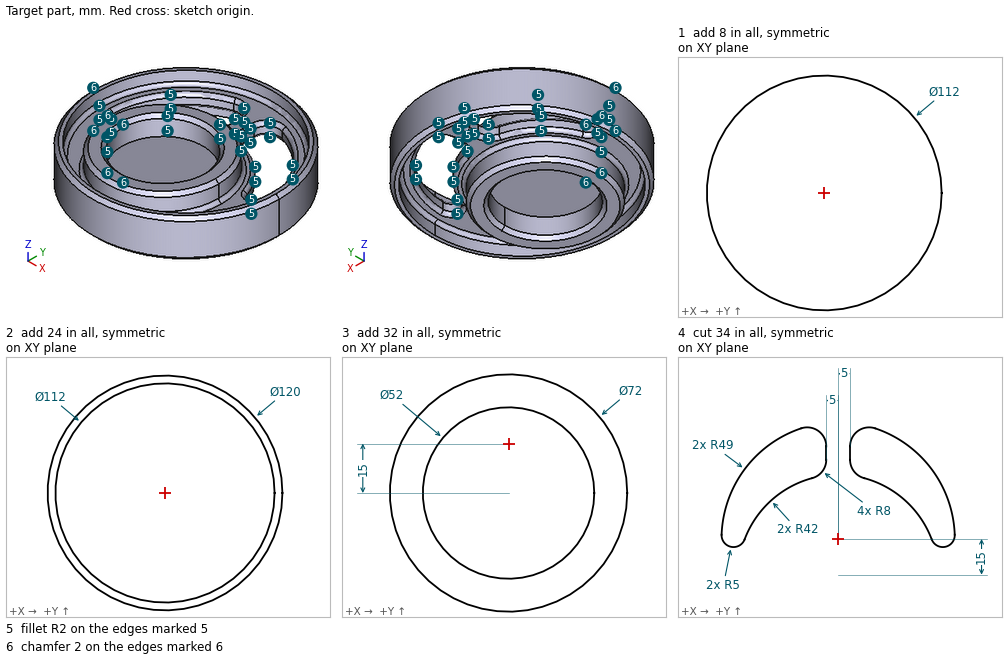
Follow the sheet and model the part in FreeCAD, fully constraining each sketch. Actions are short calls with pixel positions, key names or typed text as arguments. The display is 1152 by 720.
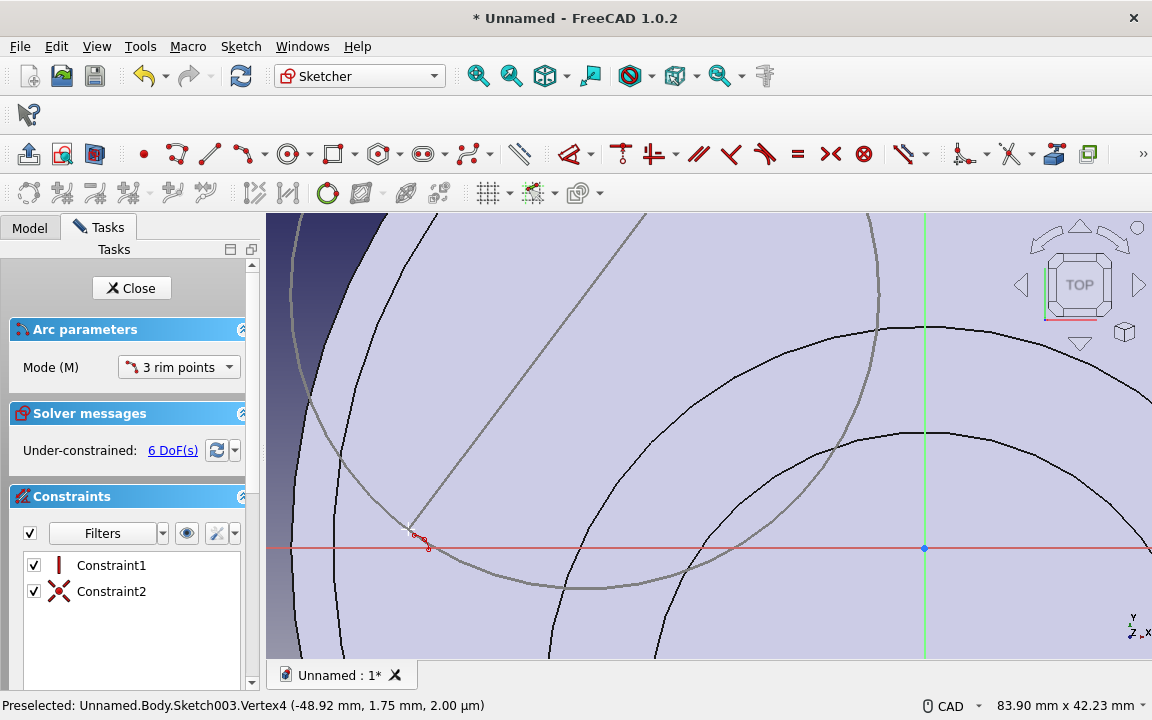
scroll(409, 530, down, 4)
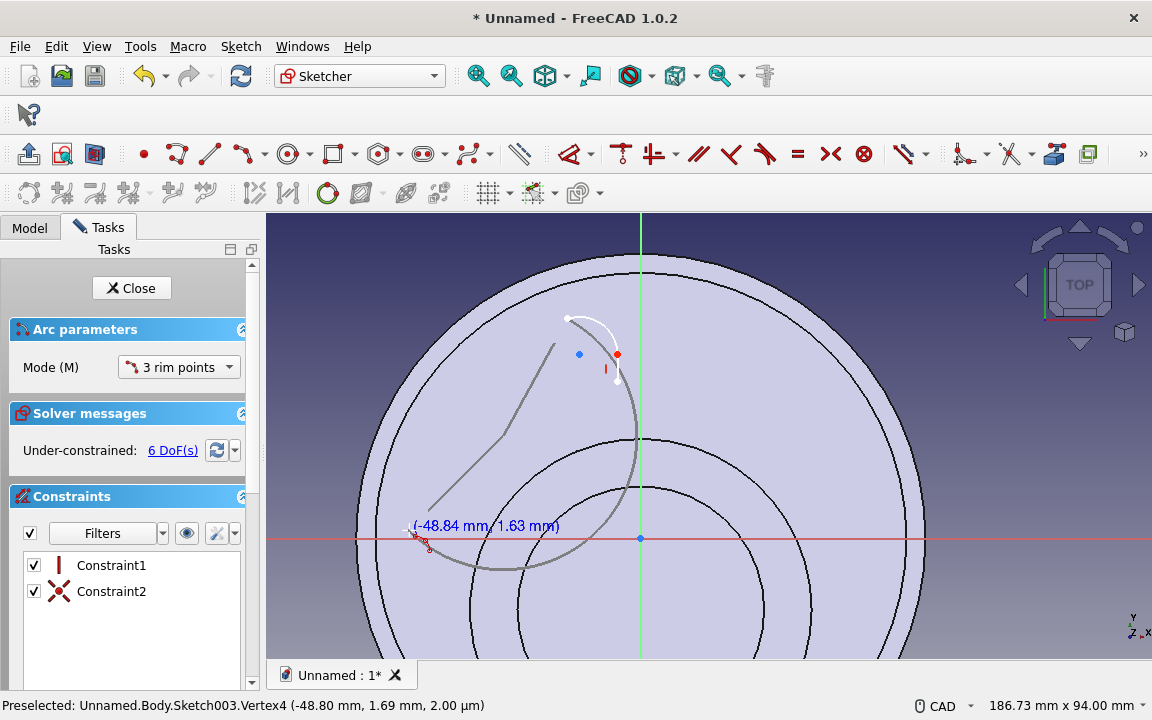
click(455, 399)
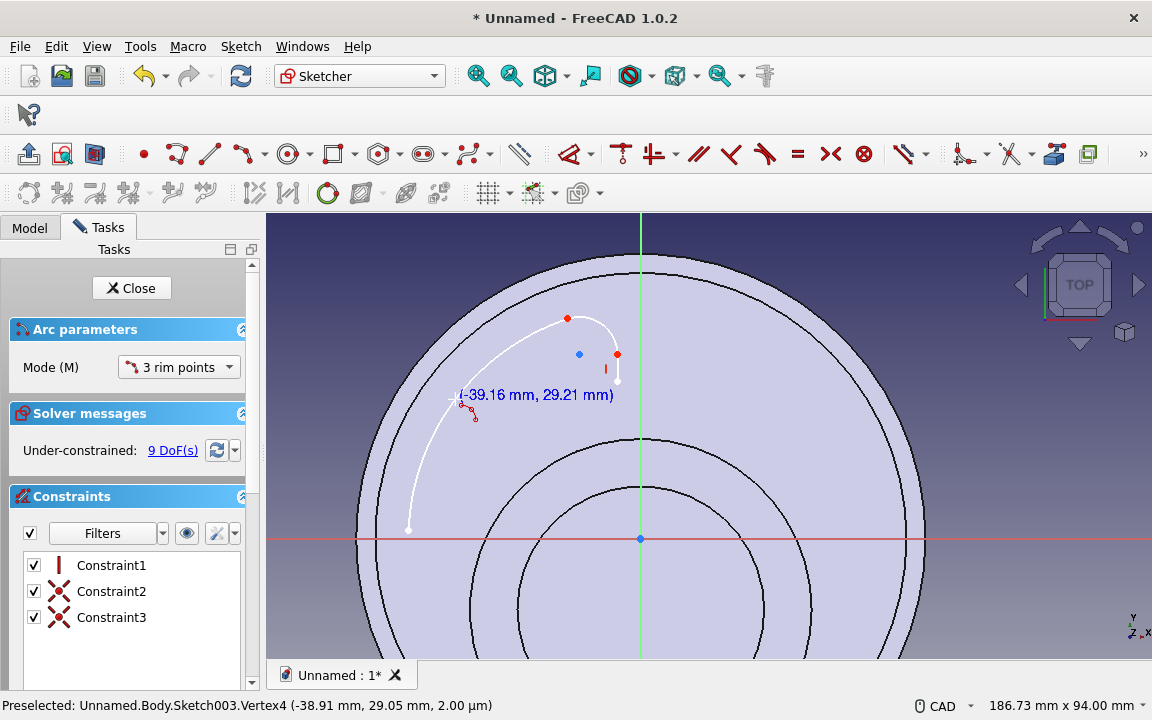
scroll(408, 530, up, 4)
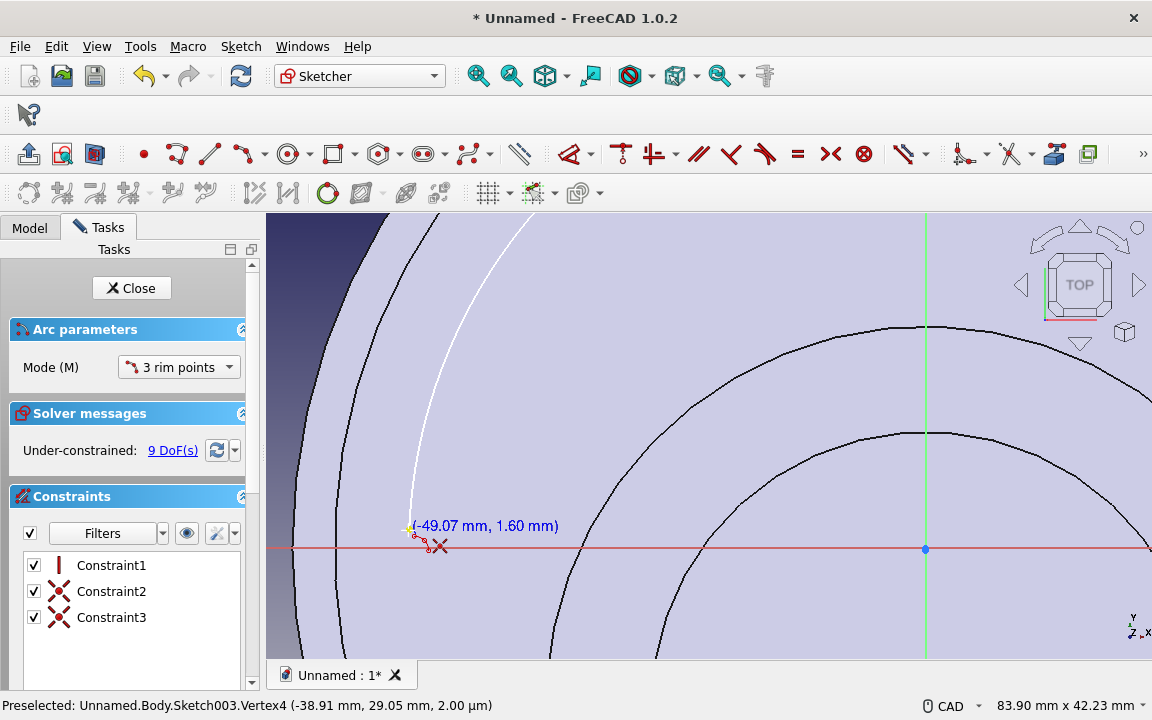
click(409, 530)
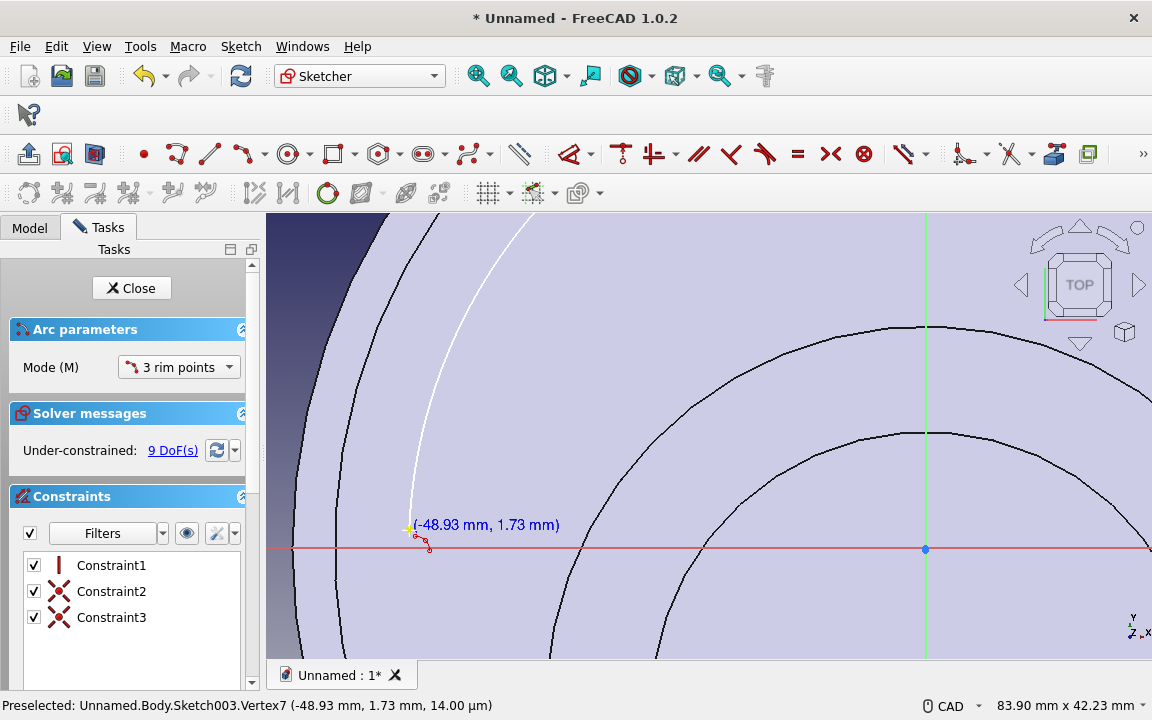
scroll(511, 550, up, 12)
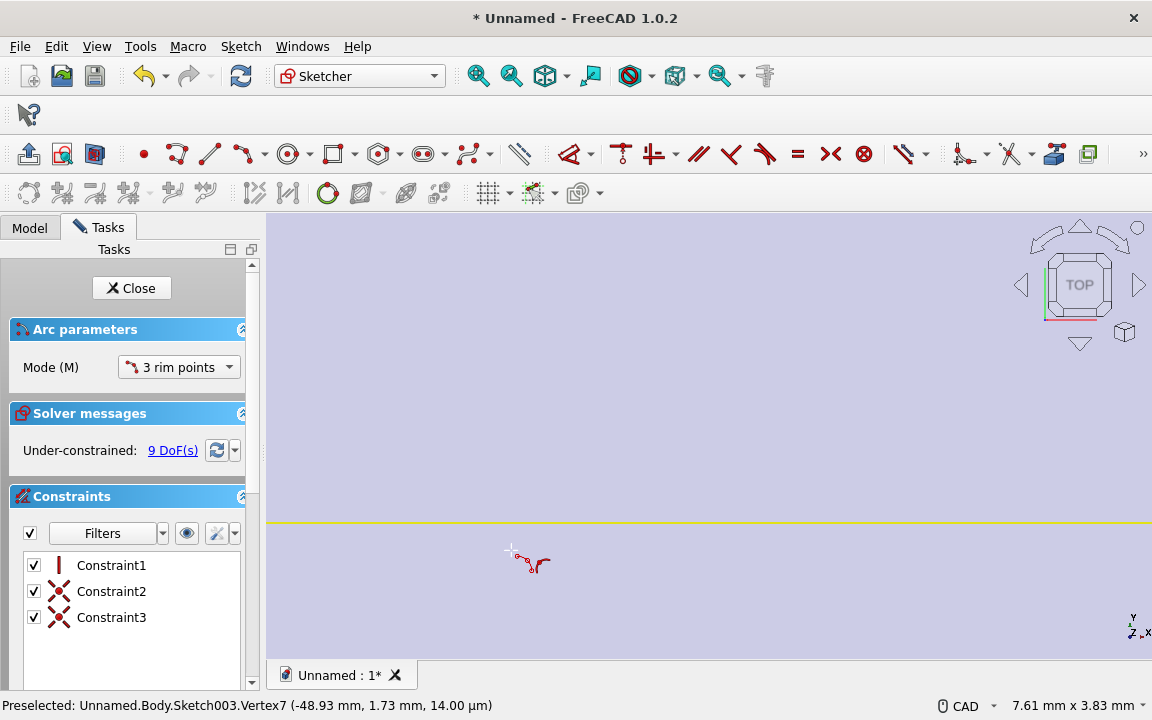
click(509, 542)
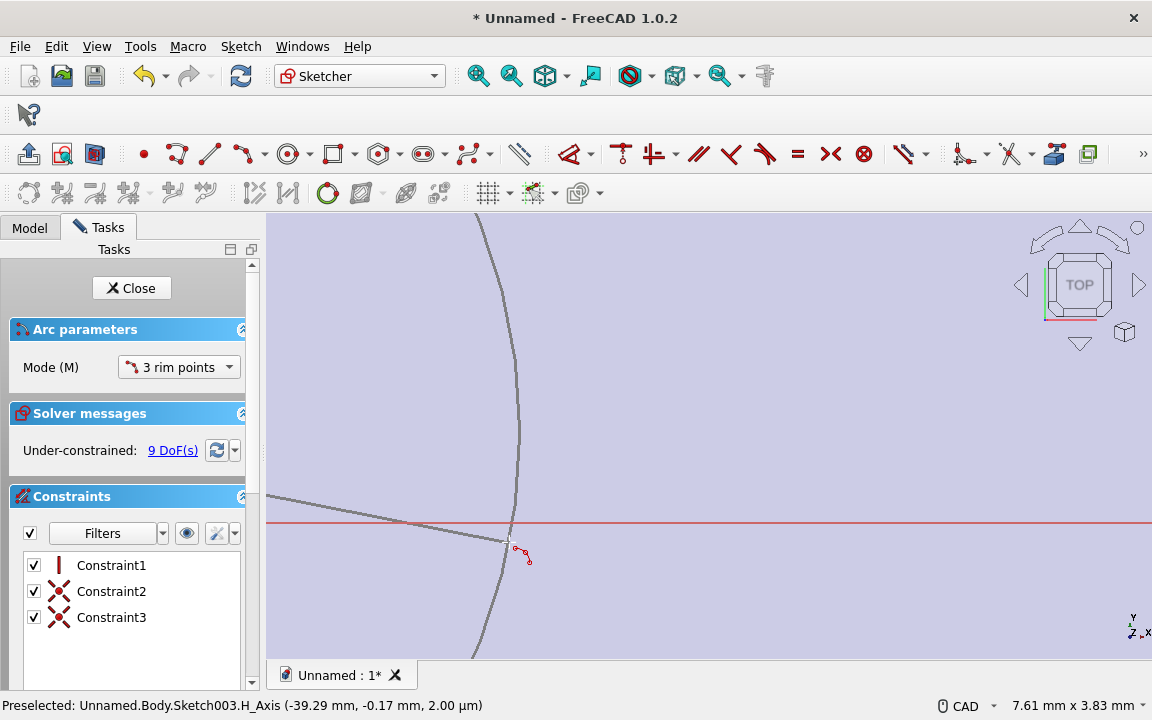
scroll(408, 563, down, 15)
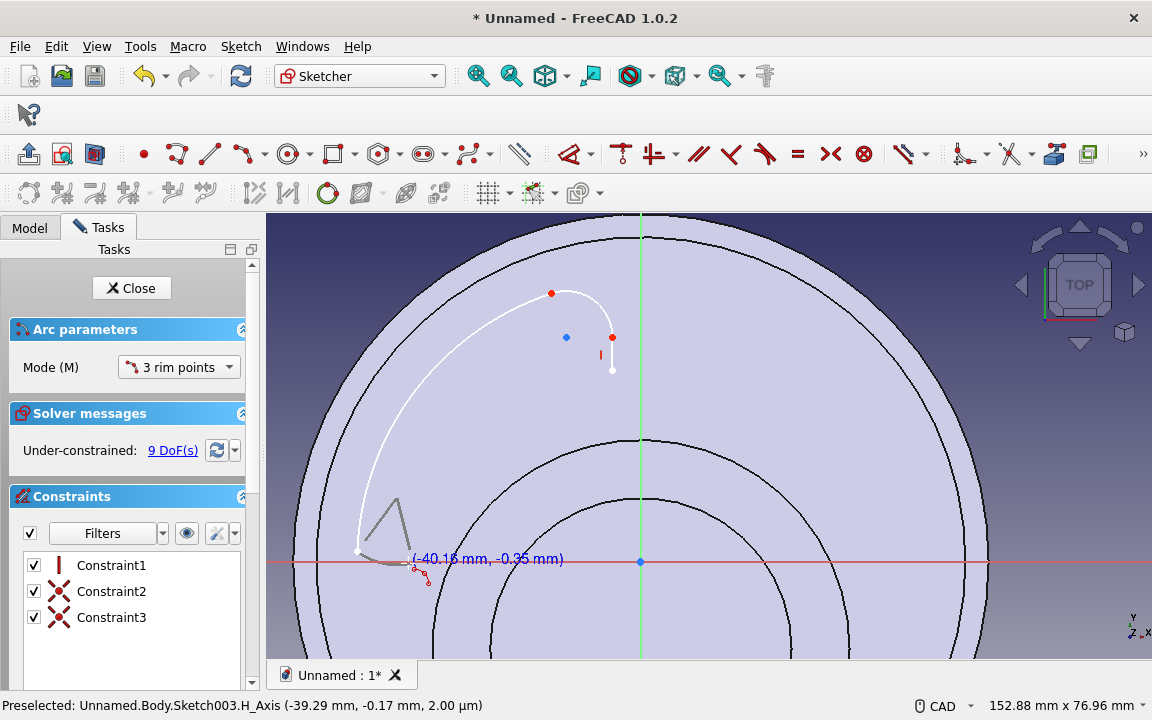
click(380, 581)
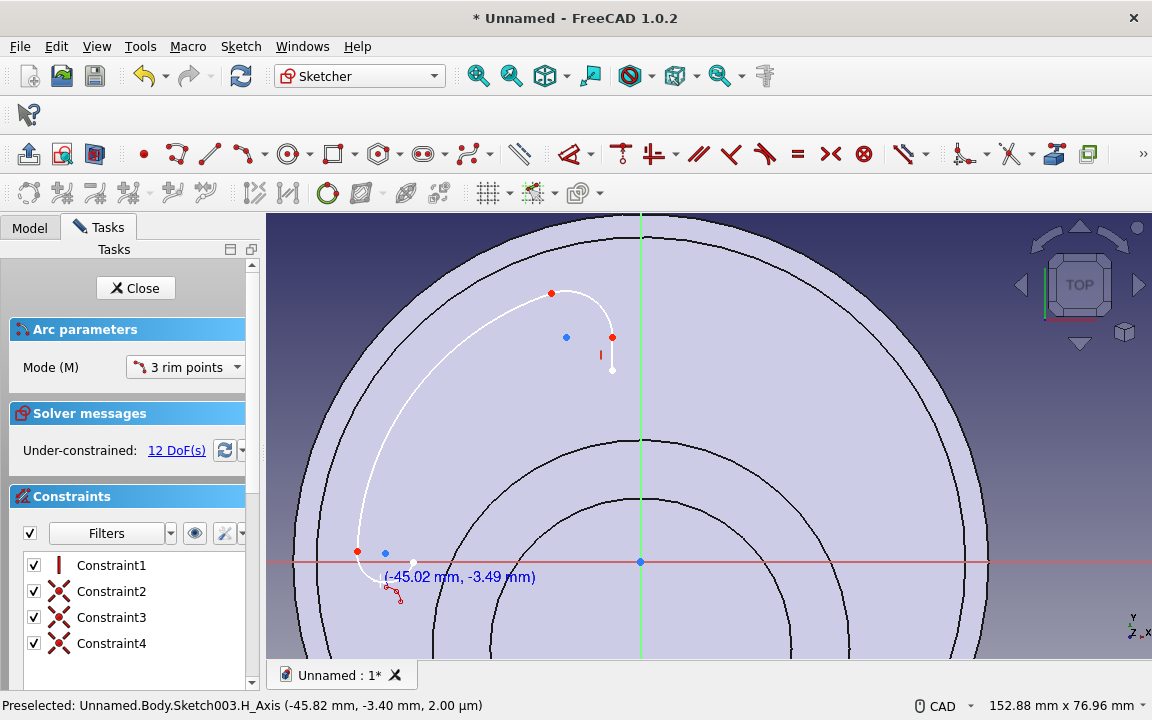
scroll(413, 563, up, 15)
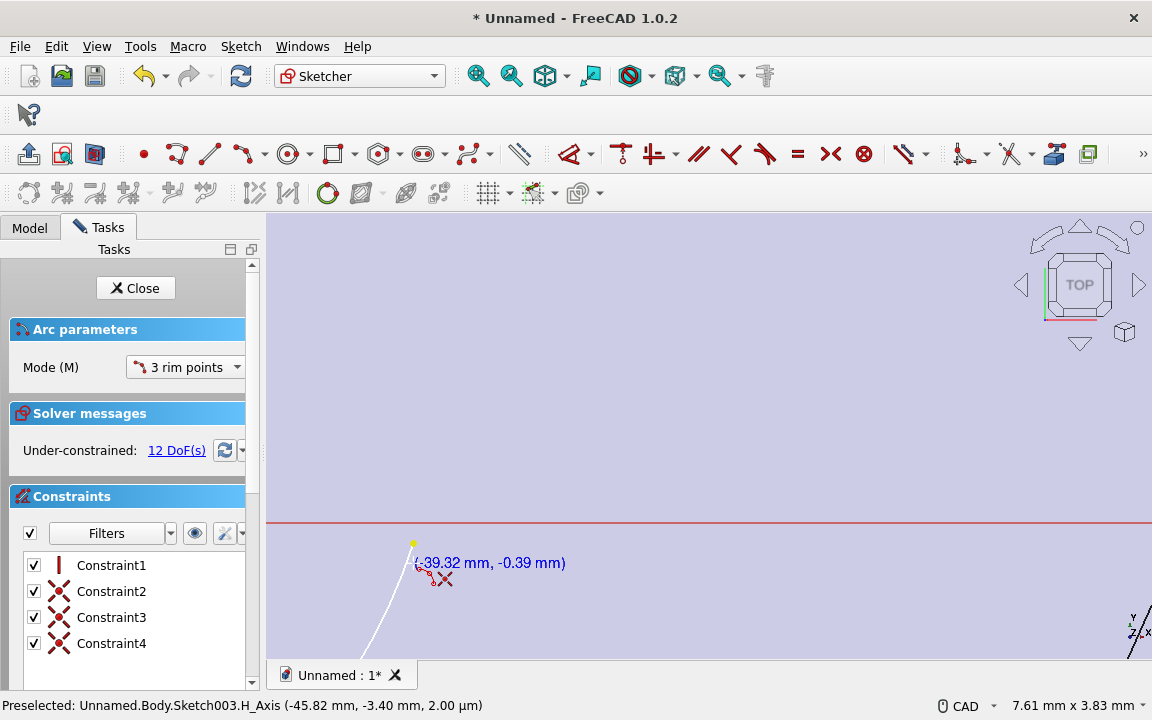
click(413, 543)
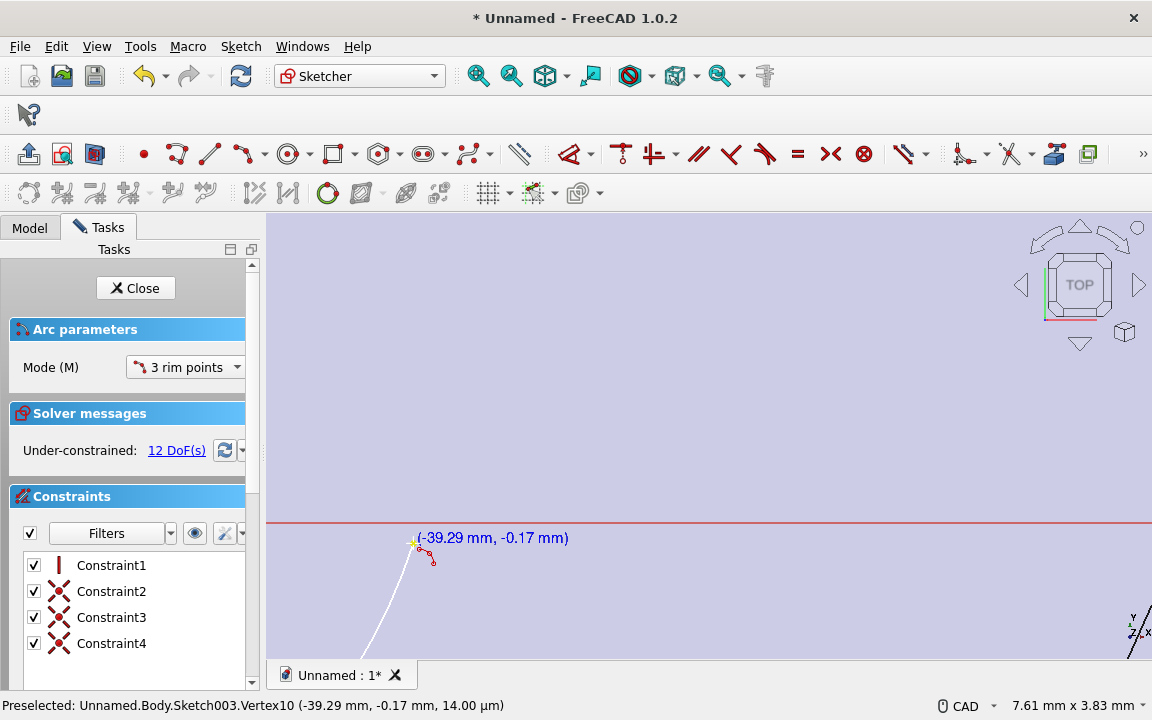
scroll(413, 563, down, 15)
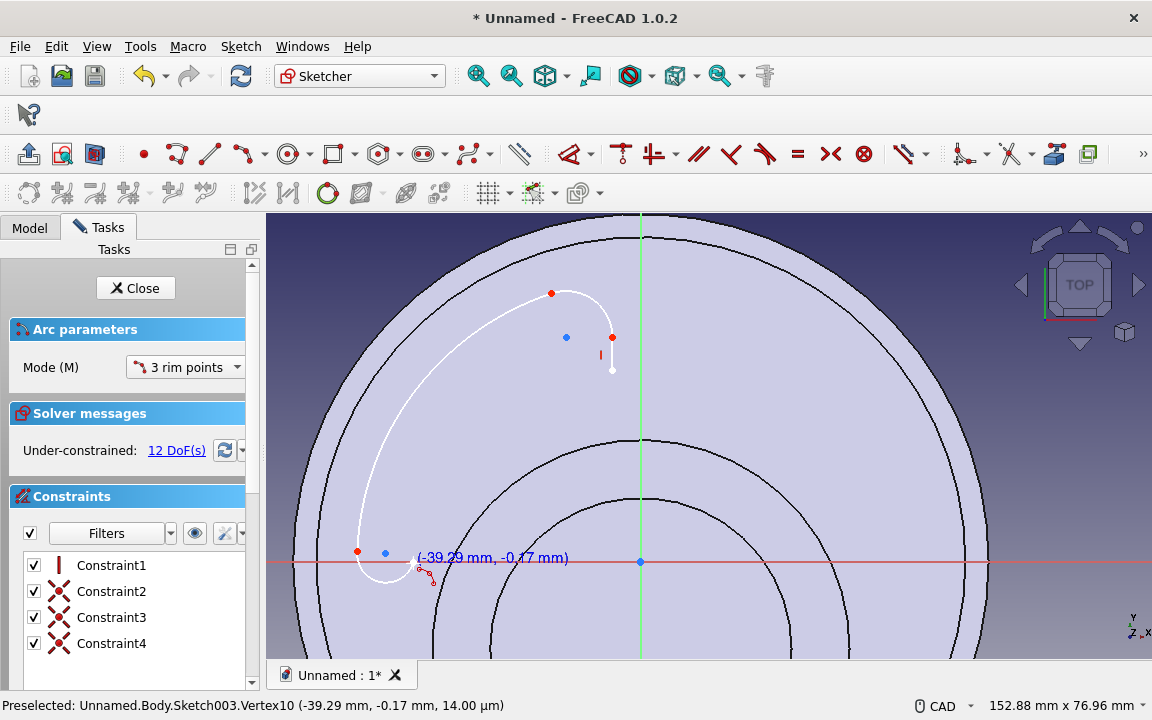
click(578, 414)
click(477, 468)